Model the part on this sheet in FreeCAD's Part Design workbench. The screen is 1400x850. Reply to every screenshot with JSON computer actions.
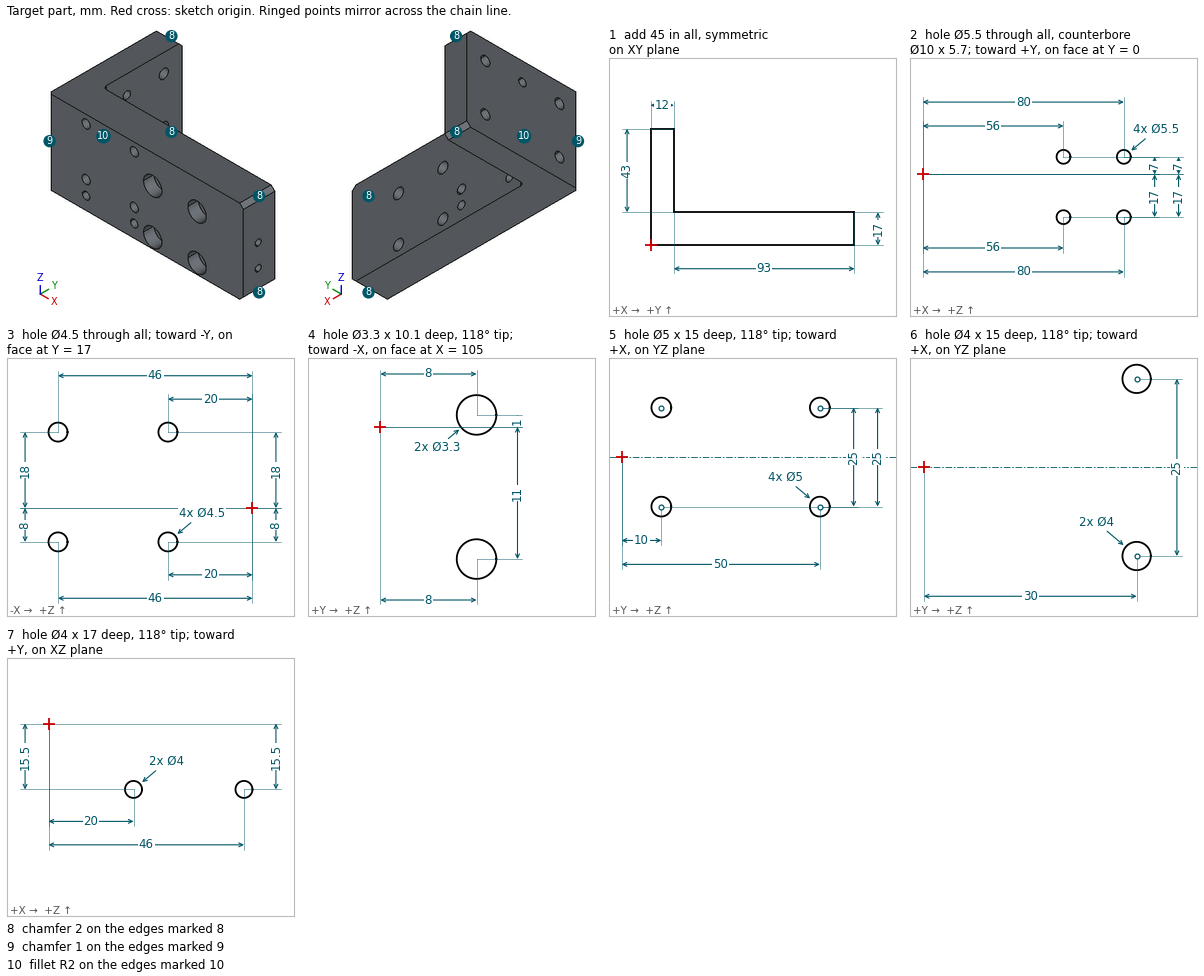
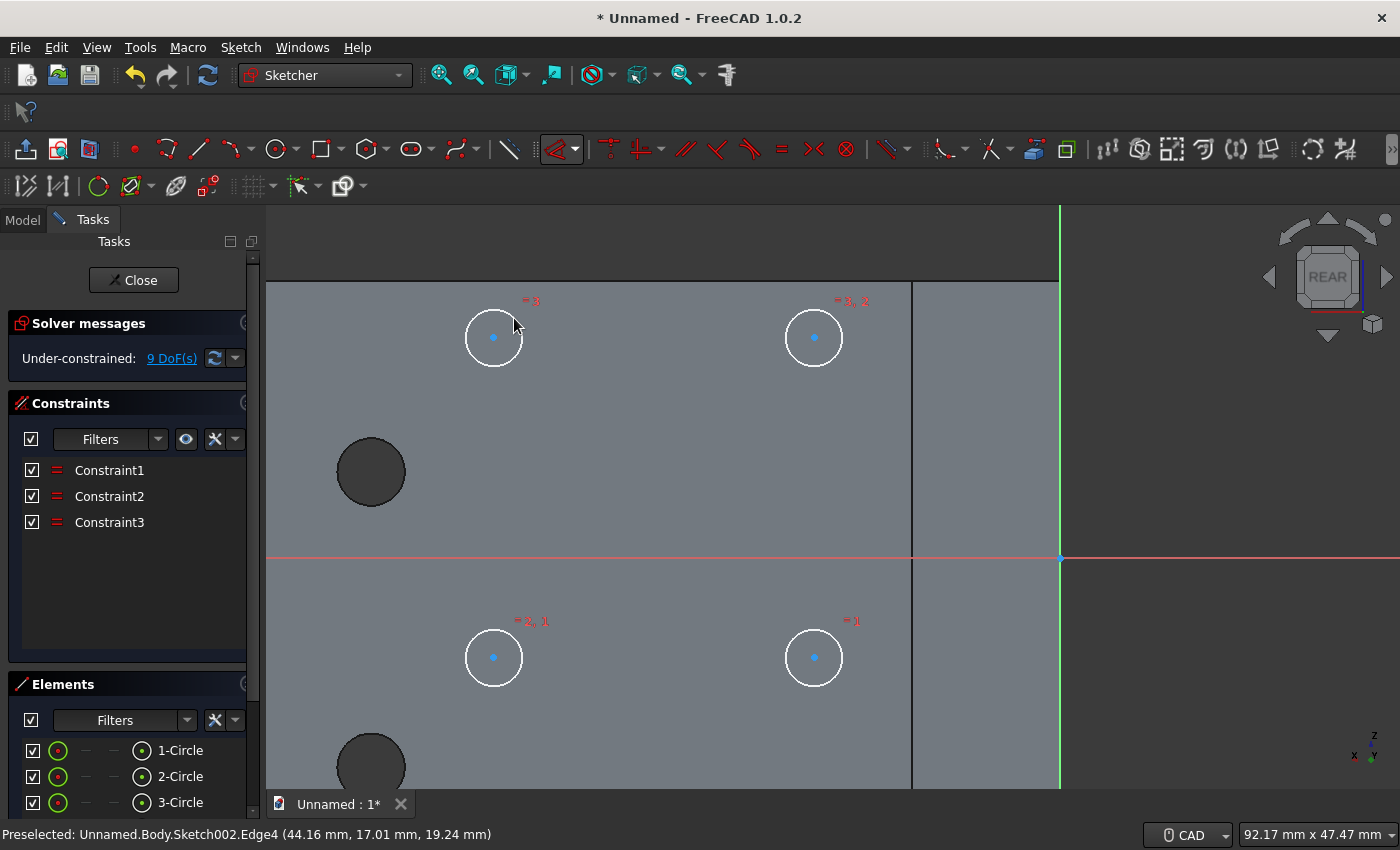
{"action": "left_click", "coordinate": [834, 638]}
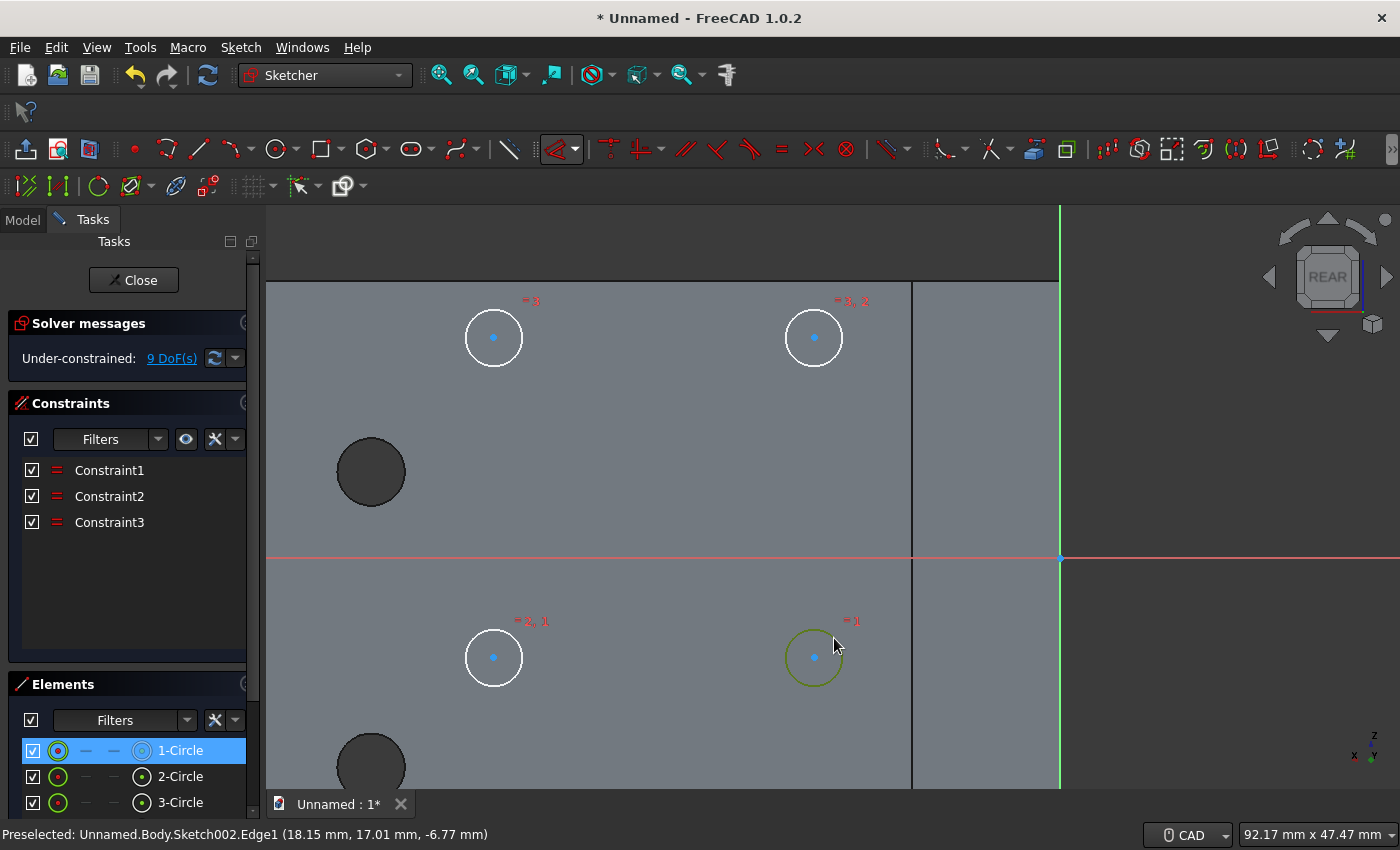
{"action": "key", "text": "k o"}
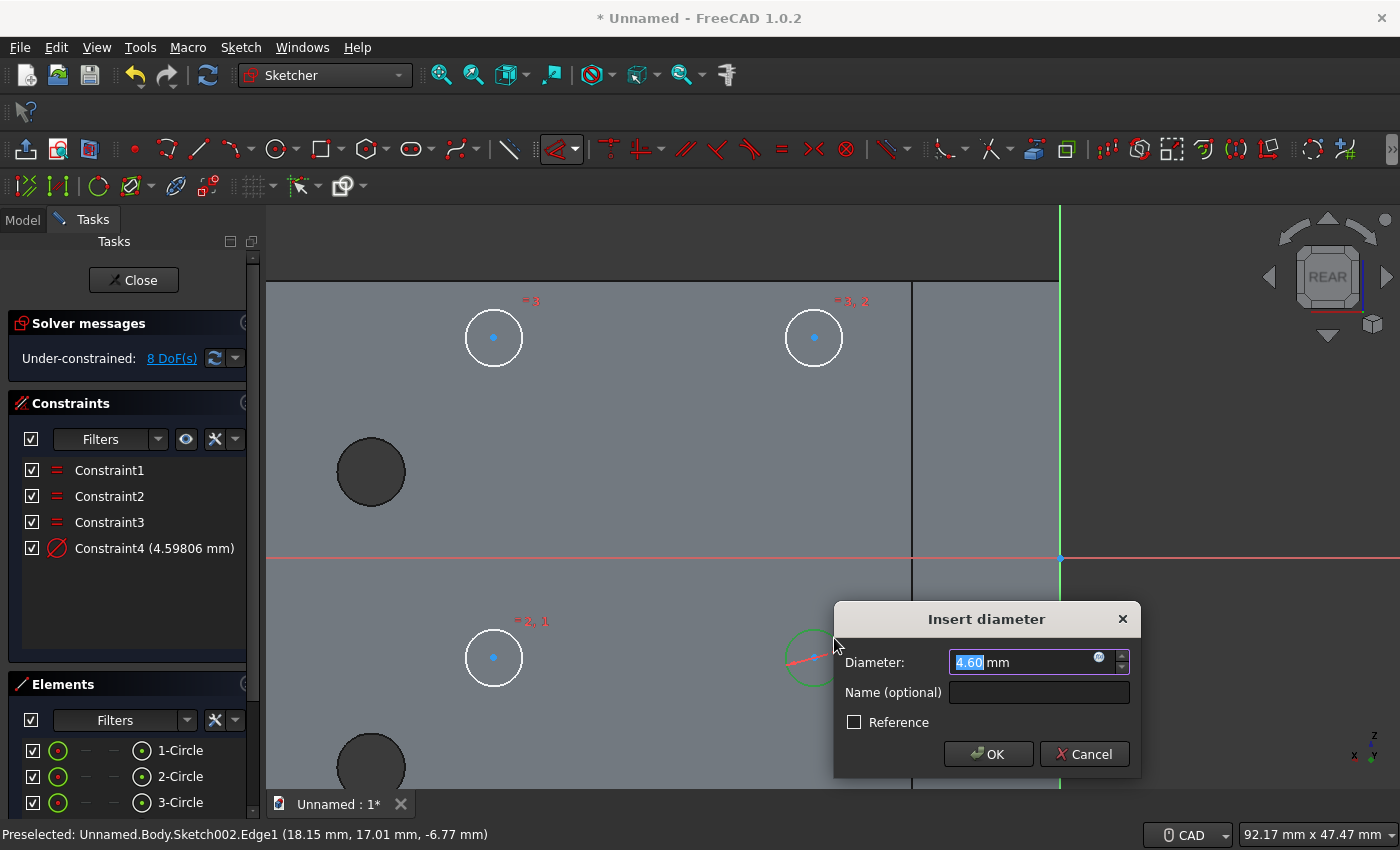
{"action": "type", "text": "4.5"}
{"action": "key", "text": "Return"}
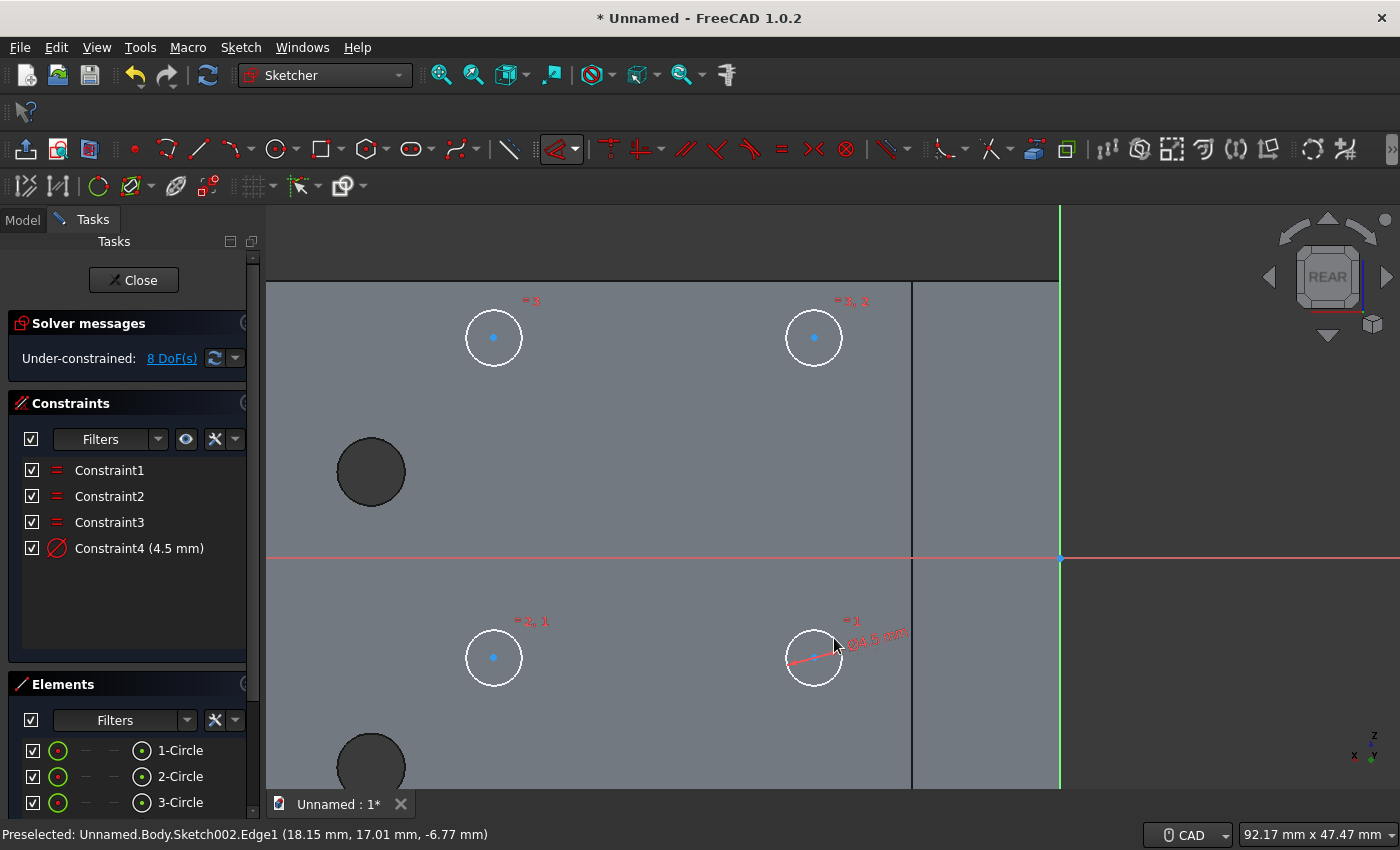
{"action": "left_click", "coordinate": [814, 658]}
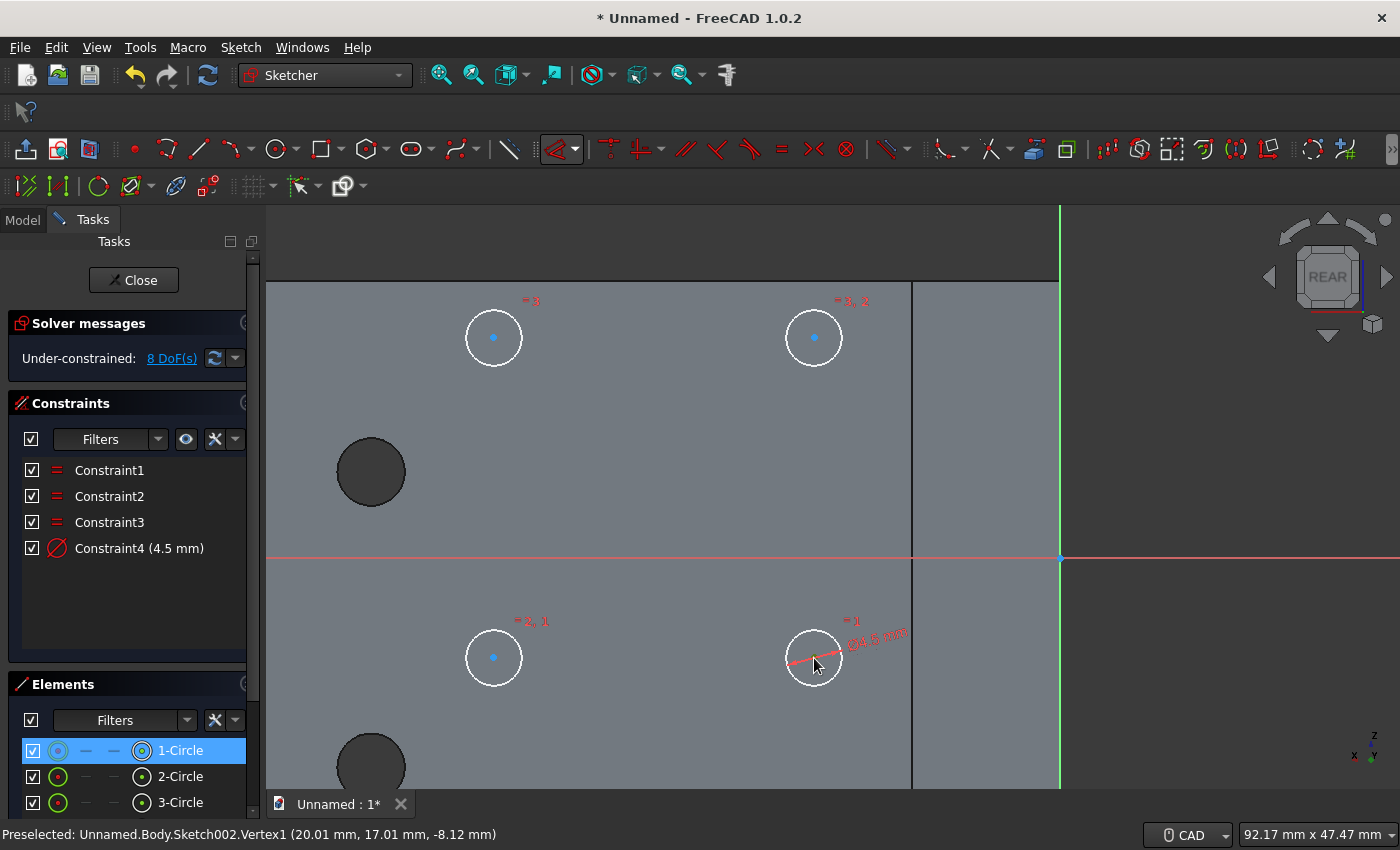
{"action": "key", "text": "i"}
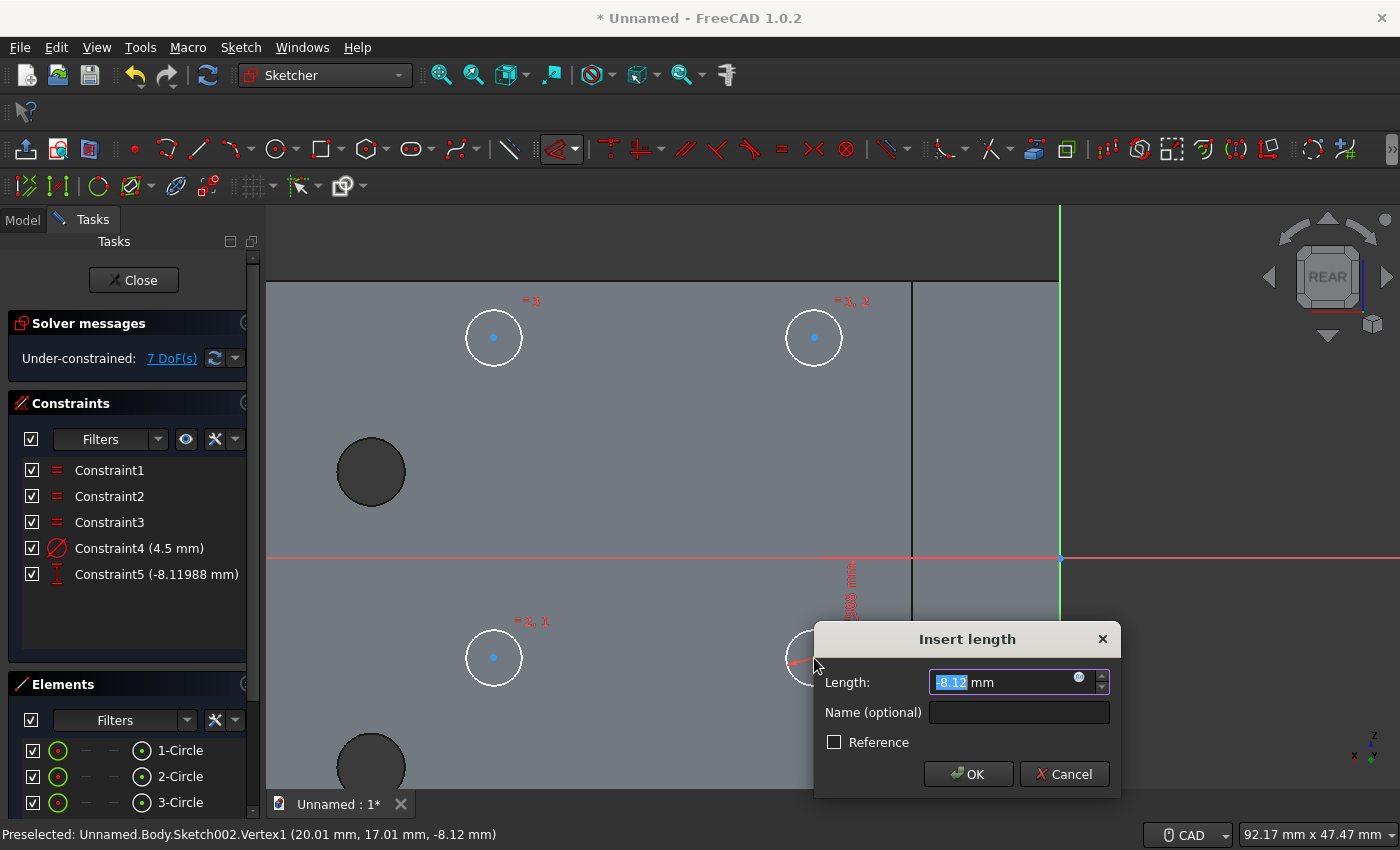
{"action": "type", "text": "-8"}
{"action": "key", "text": "Return"}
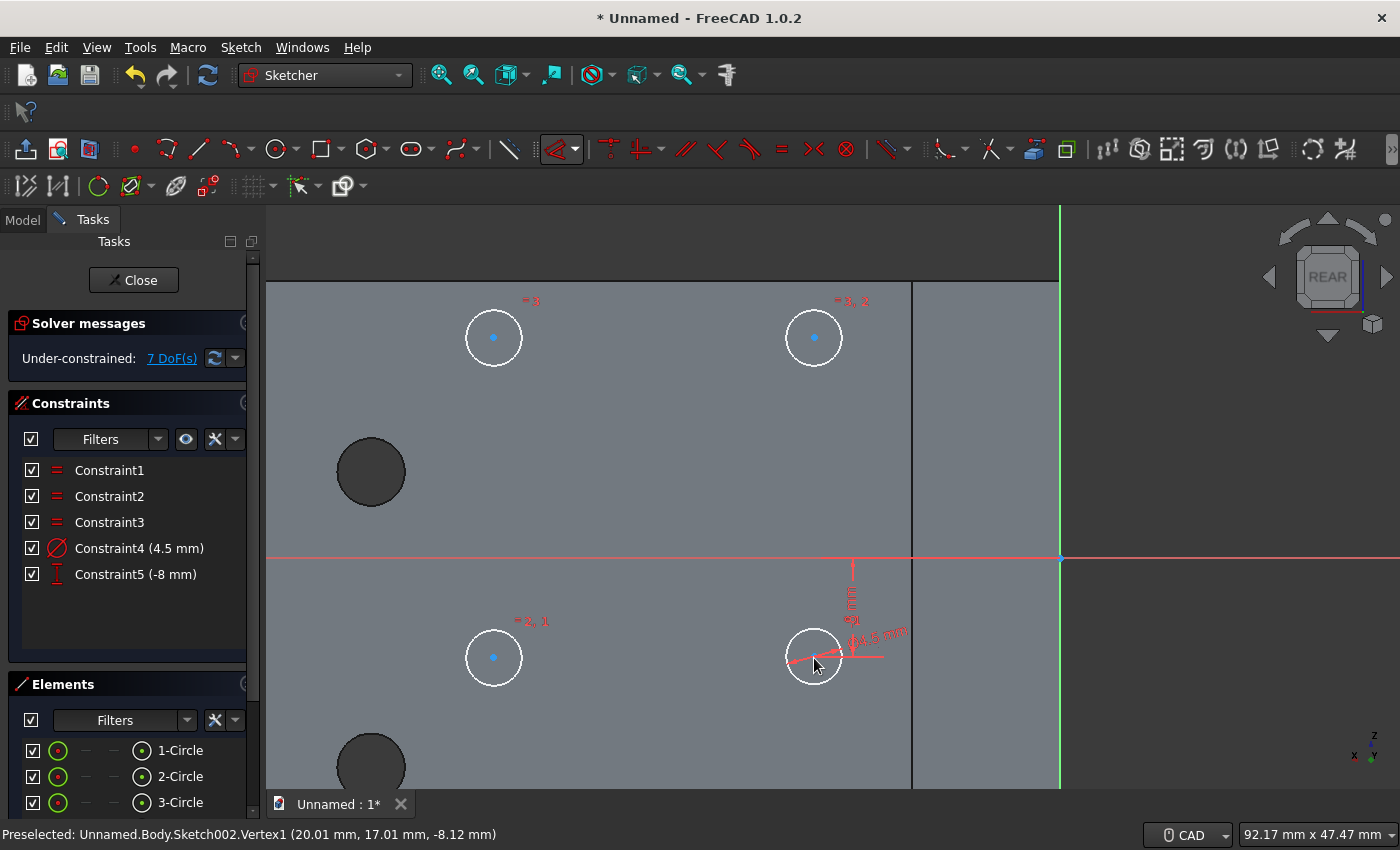
{"action": "left_click", "coordinate": [494, 658]}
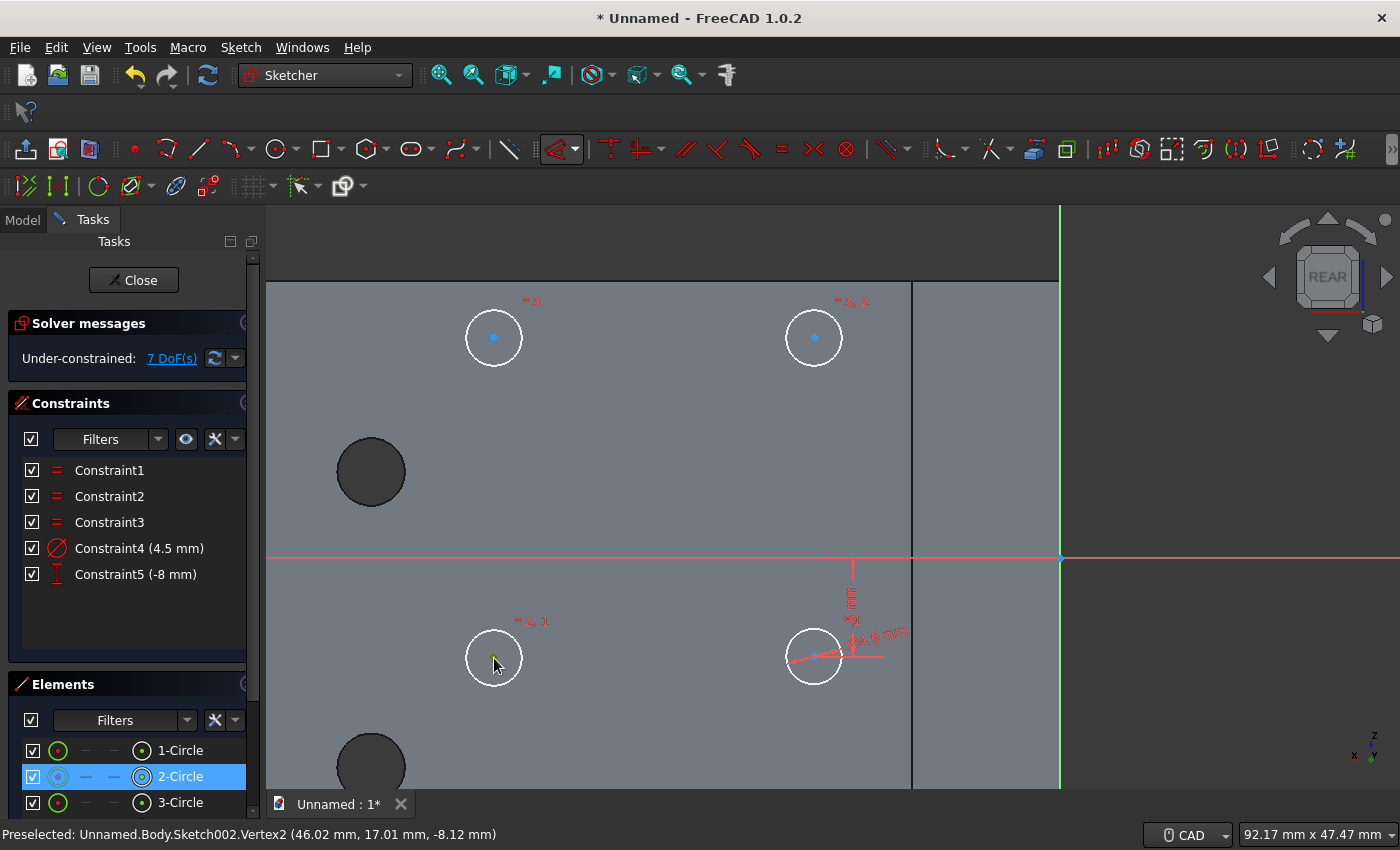
{"action": "key", "text": "i"}